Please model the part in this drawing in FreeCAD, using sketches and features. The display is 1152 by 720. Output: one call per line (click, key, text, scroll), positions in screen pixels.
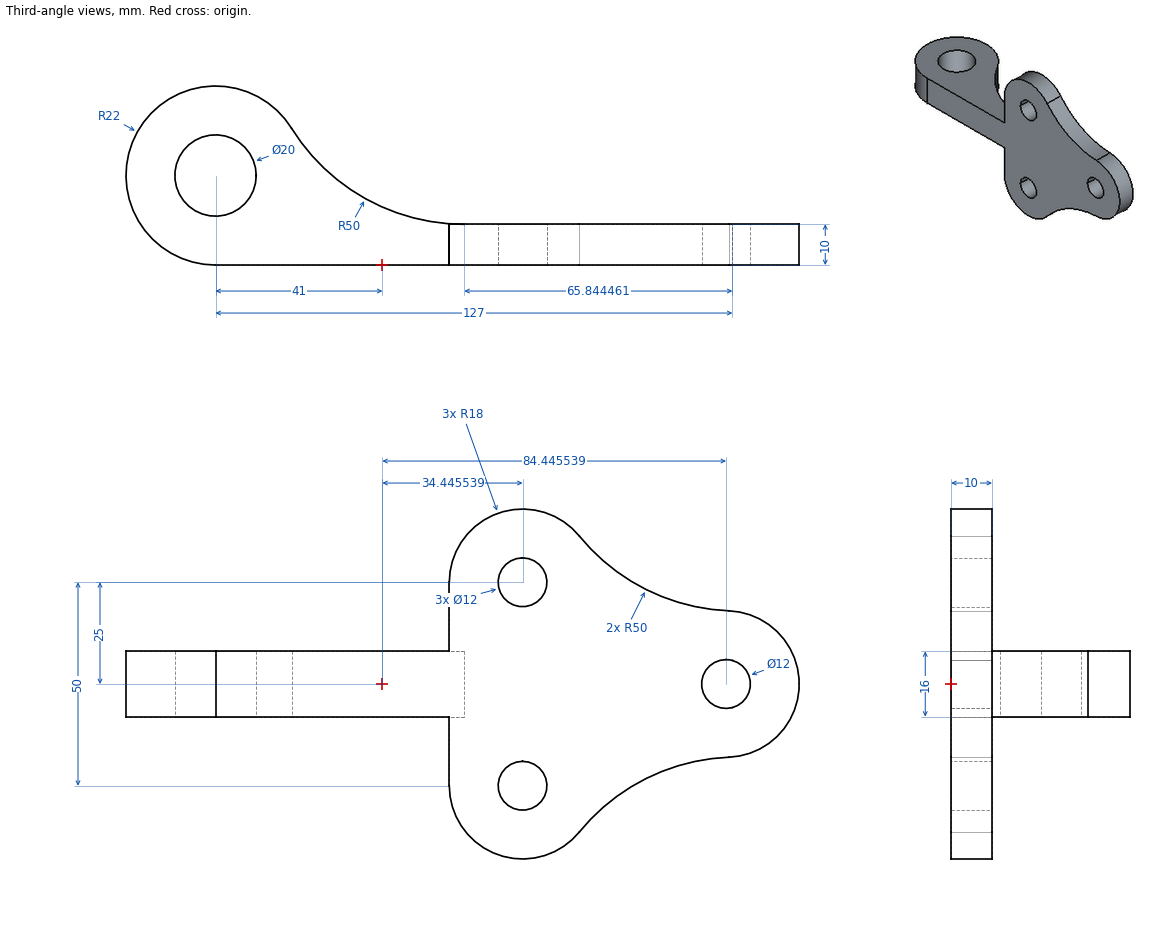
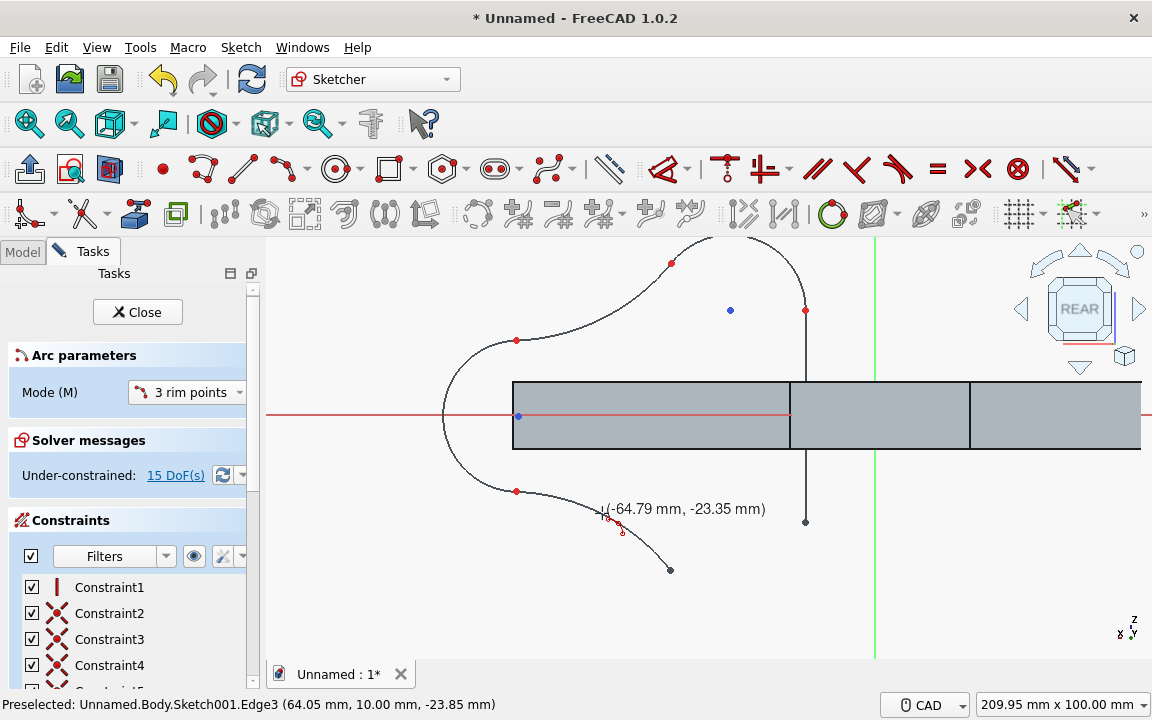
click(670, 570)
click(806, 523)
click(756, 593)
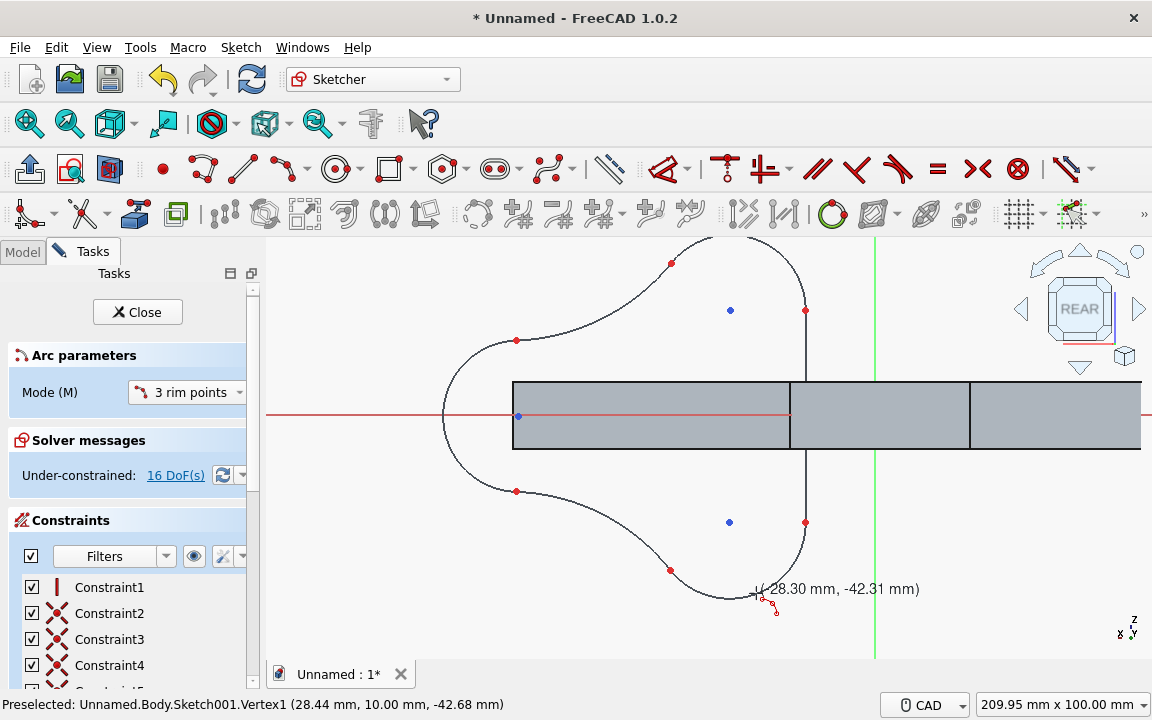
key(g)
key(c)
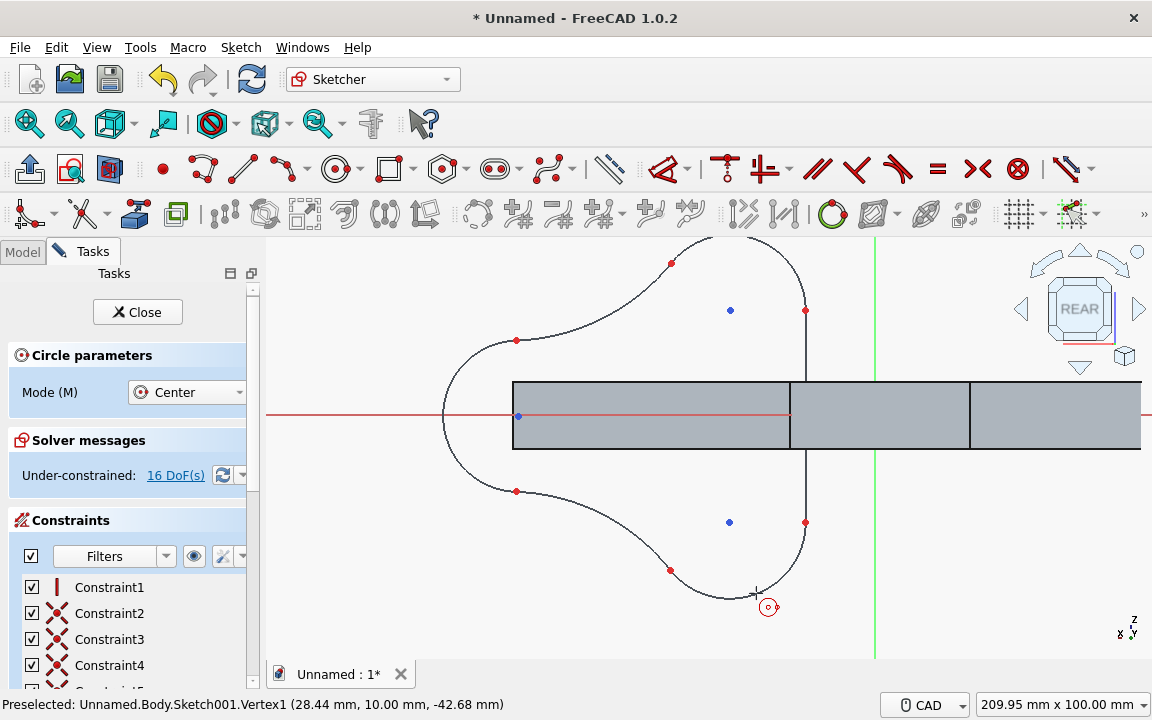
click(730, 310)
click(748, 292)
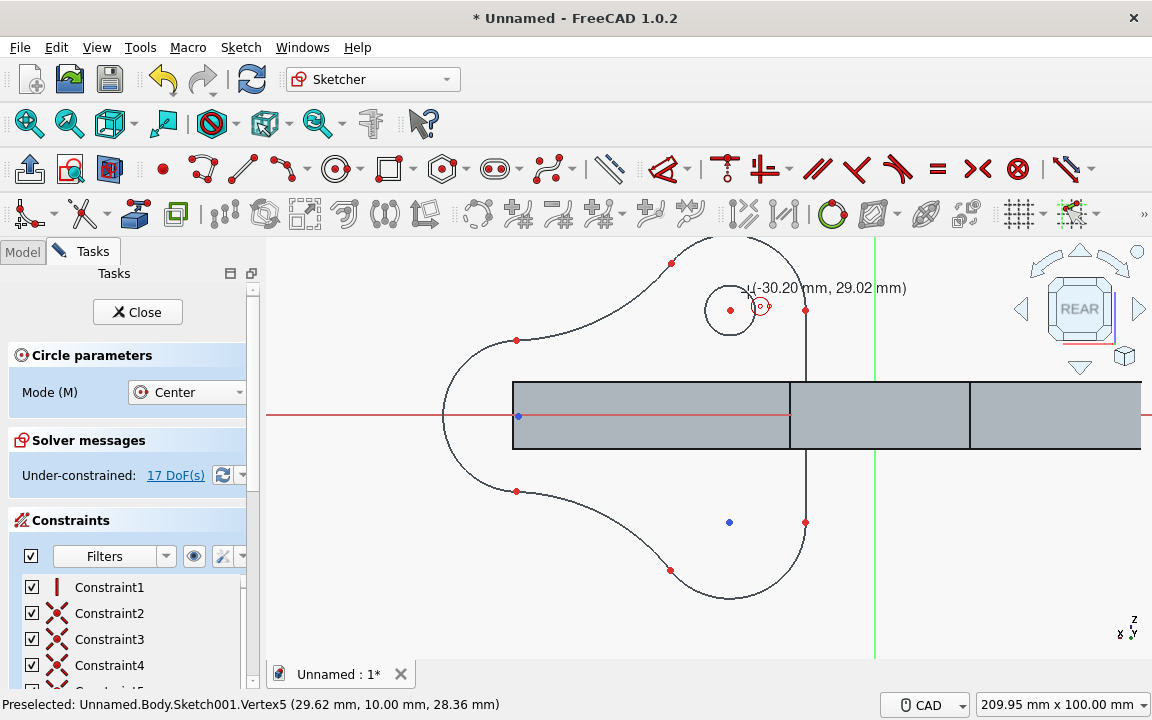
click(730, 521)
click(748, 503)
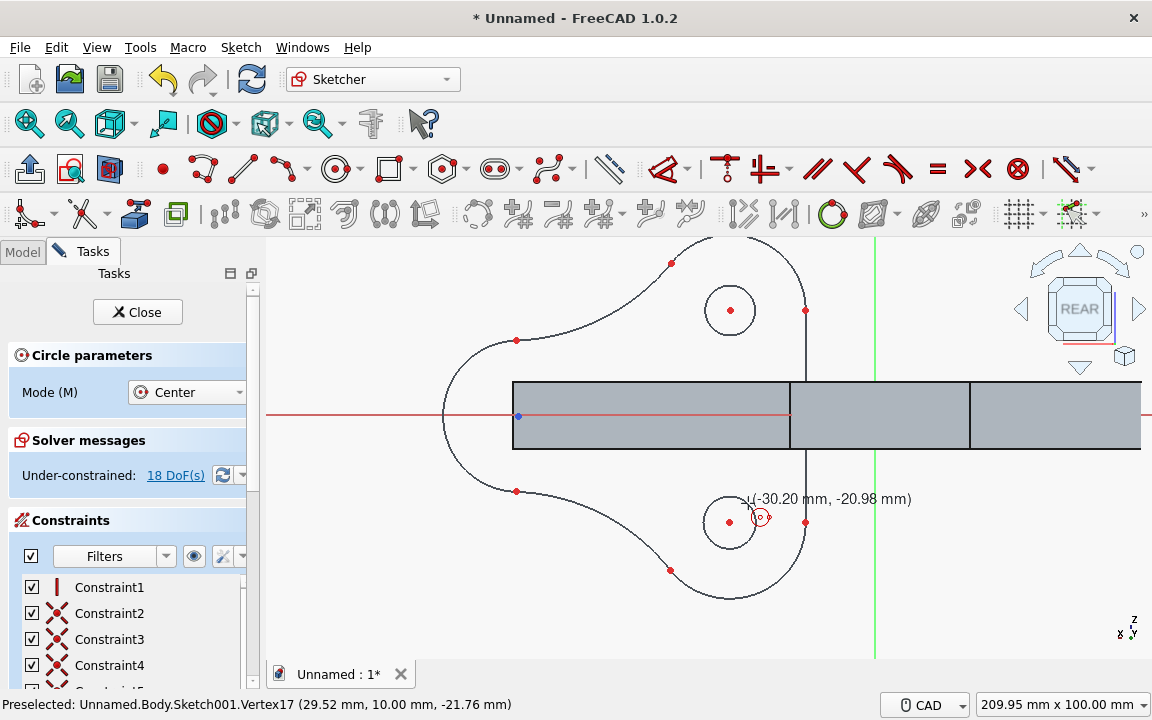
click(519, 415)
click(537, 398)
key(Escape)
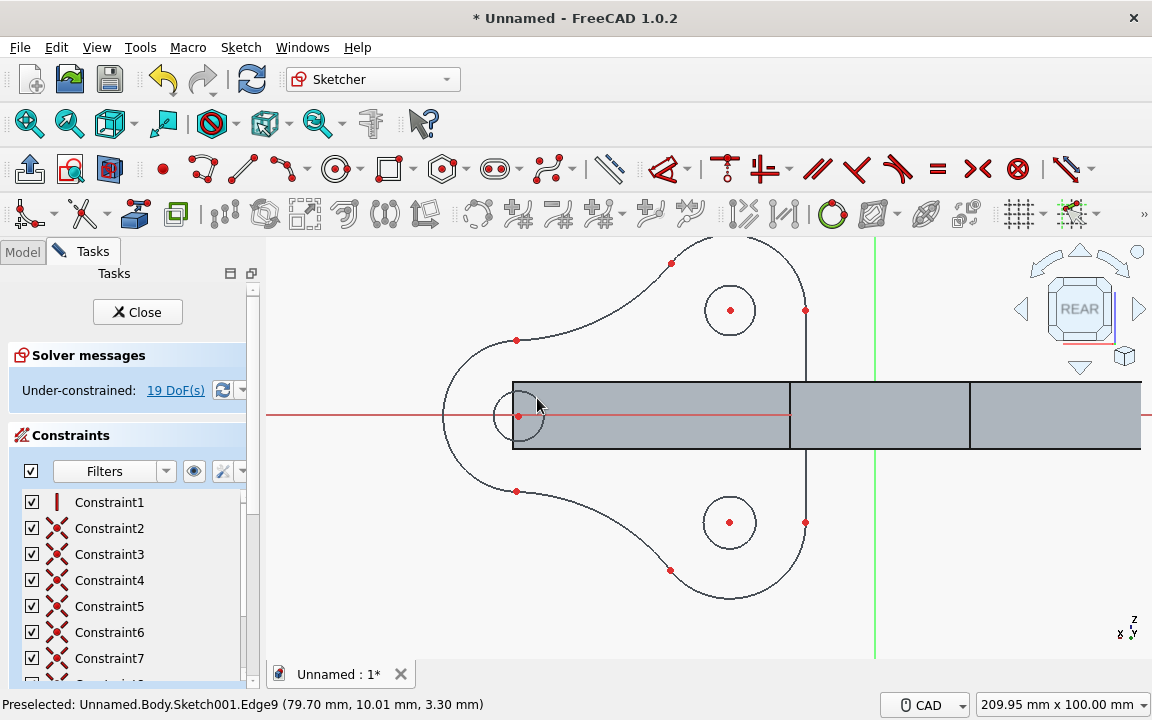
click(806, 459)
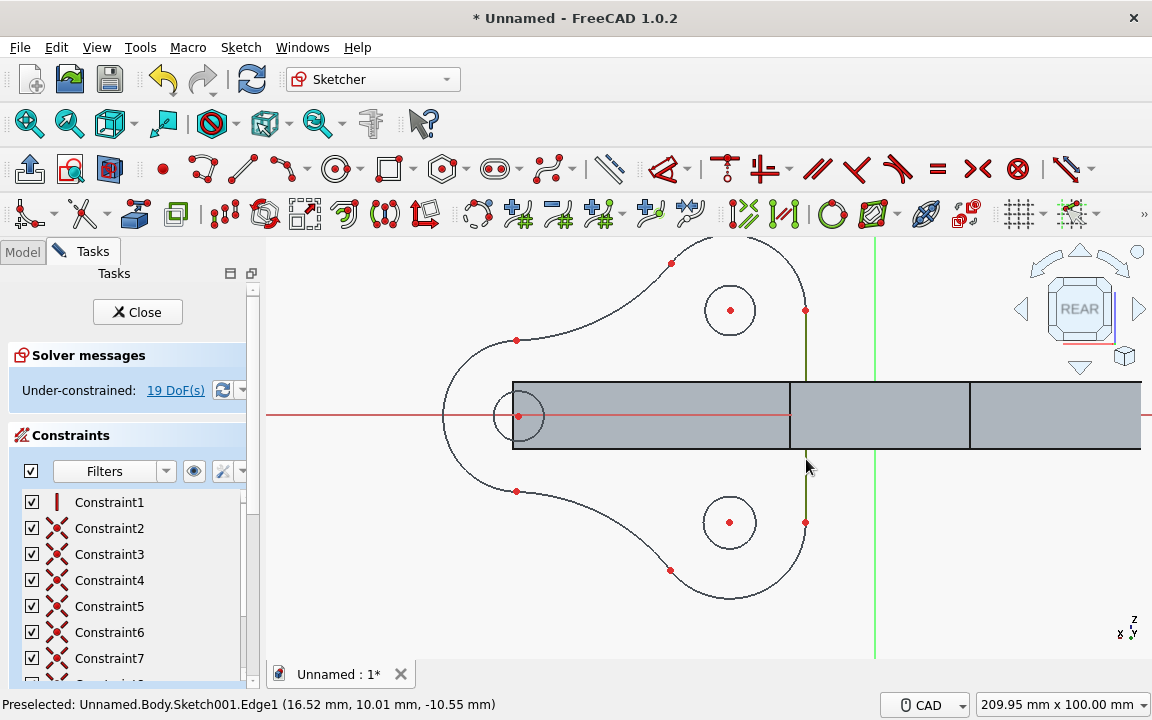
click(797, 275)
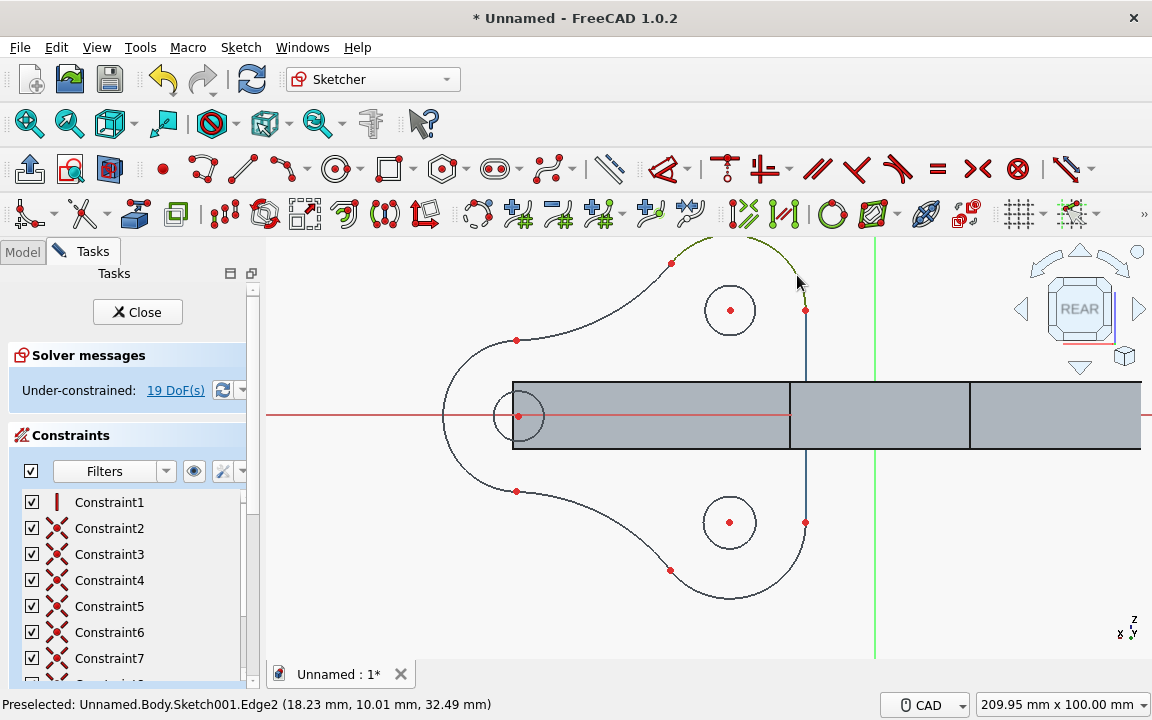
key(t)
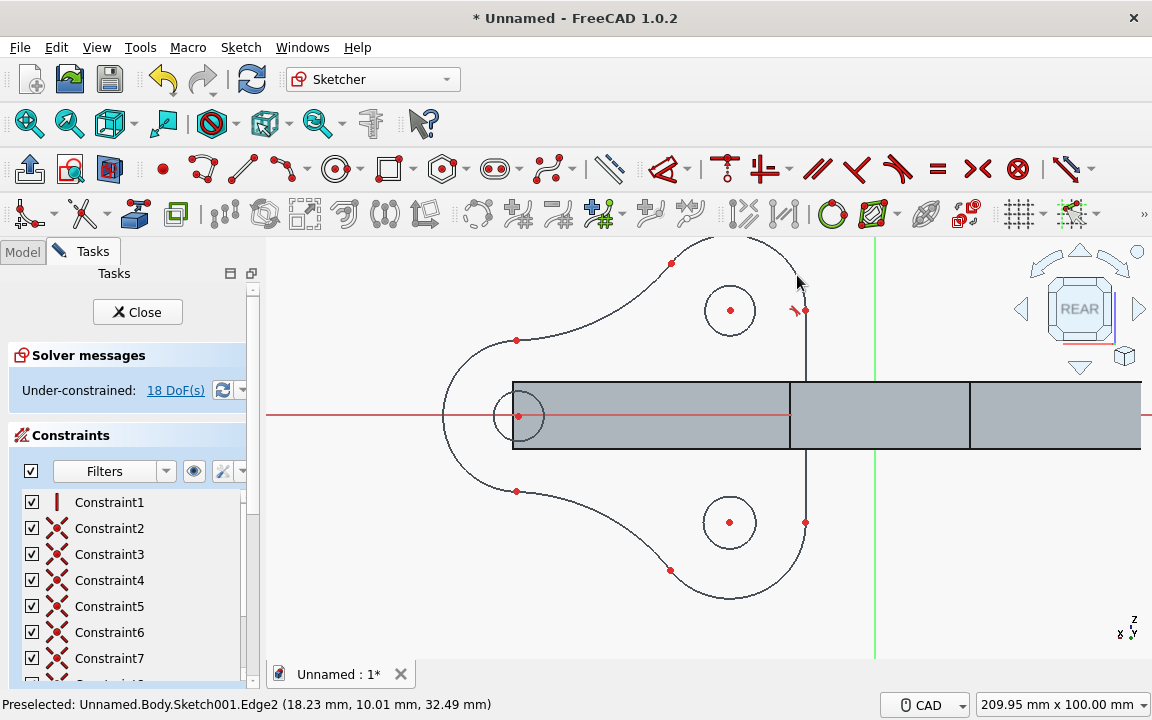
click(806, 459)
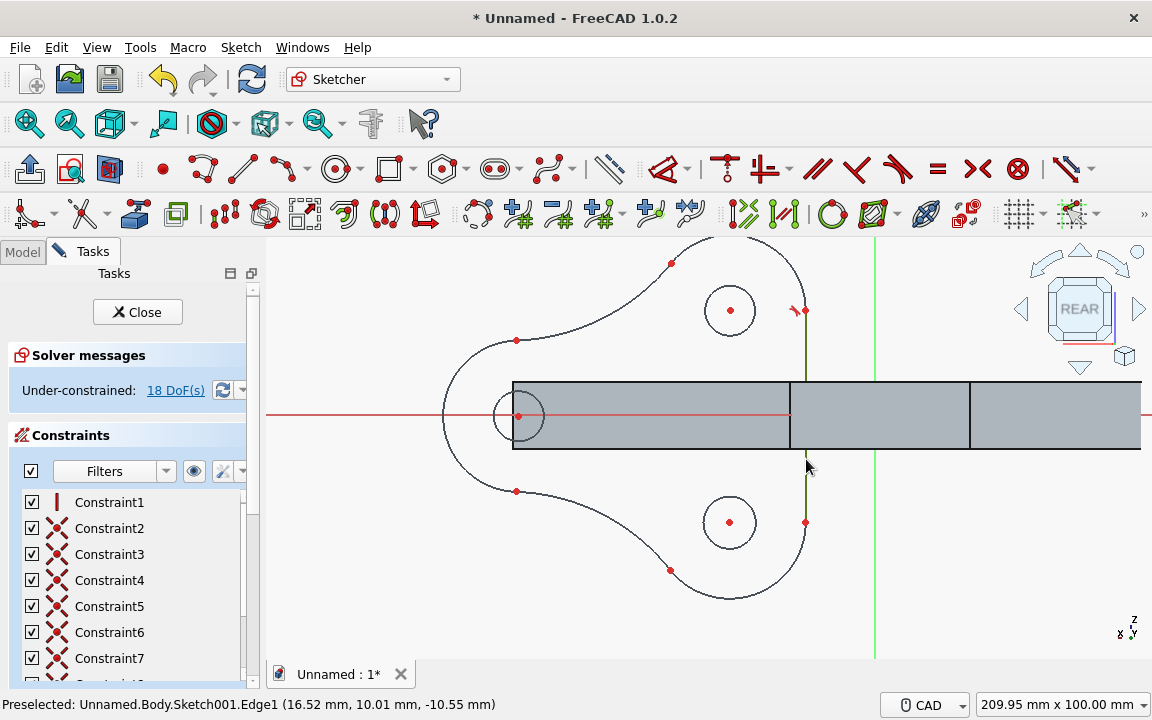
click(718, 598)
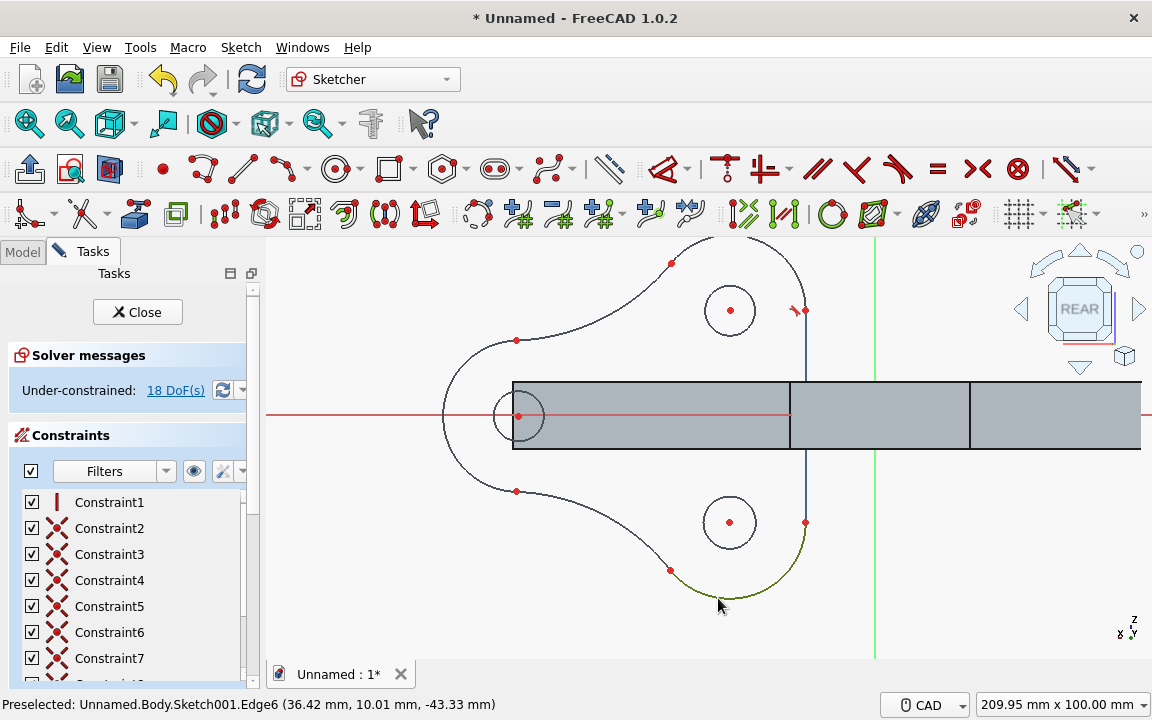
click(898, 170)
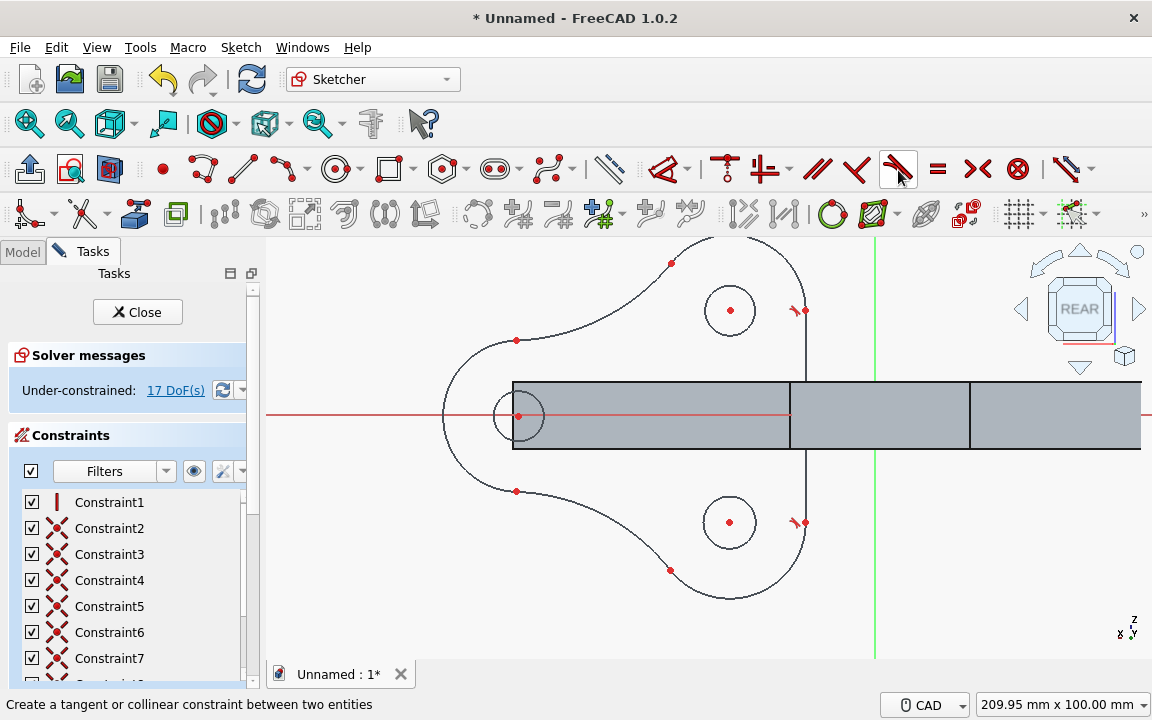
click(797, 275)